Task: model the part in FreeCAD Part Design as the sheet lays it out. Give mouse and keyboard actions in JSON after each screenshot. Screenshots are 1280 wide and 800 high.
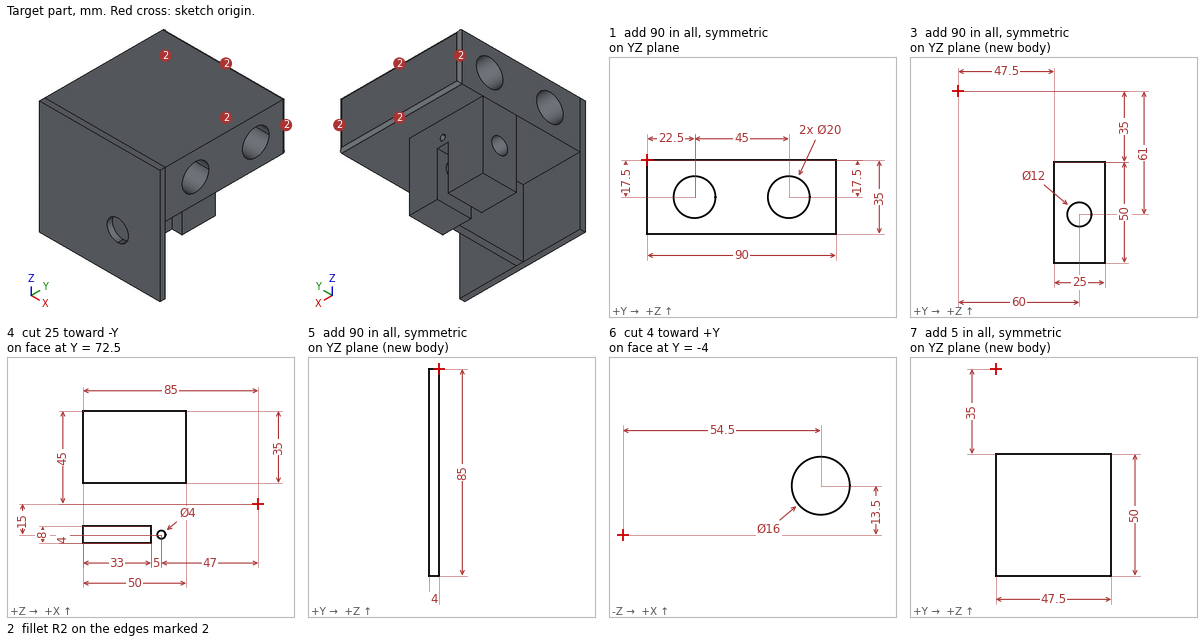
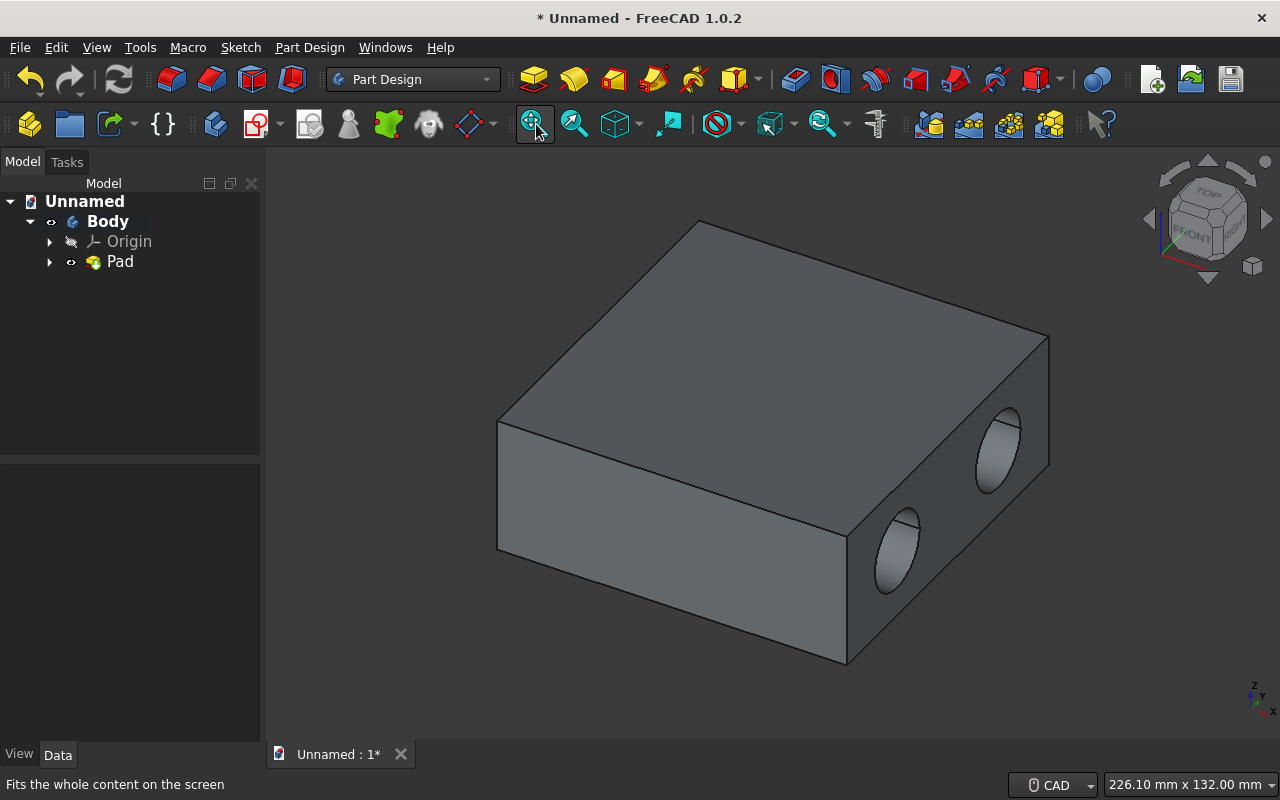
{"action": "key", "text": "0"}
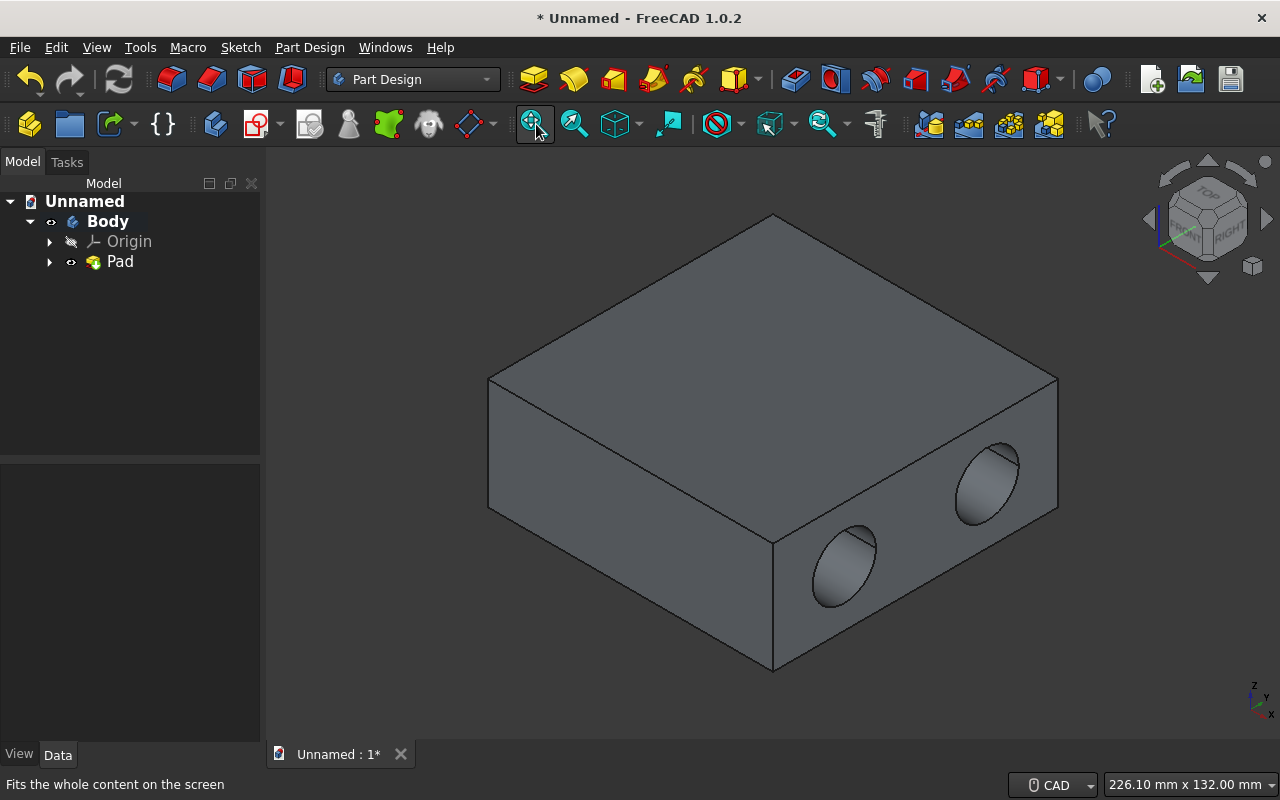
{"action": "key", "text": "2"}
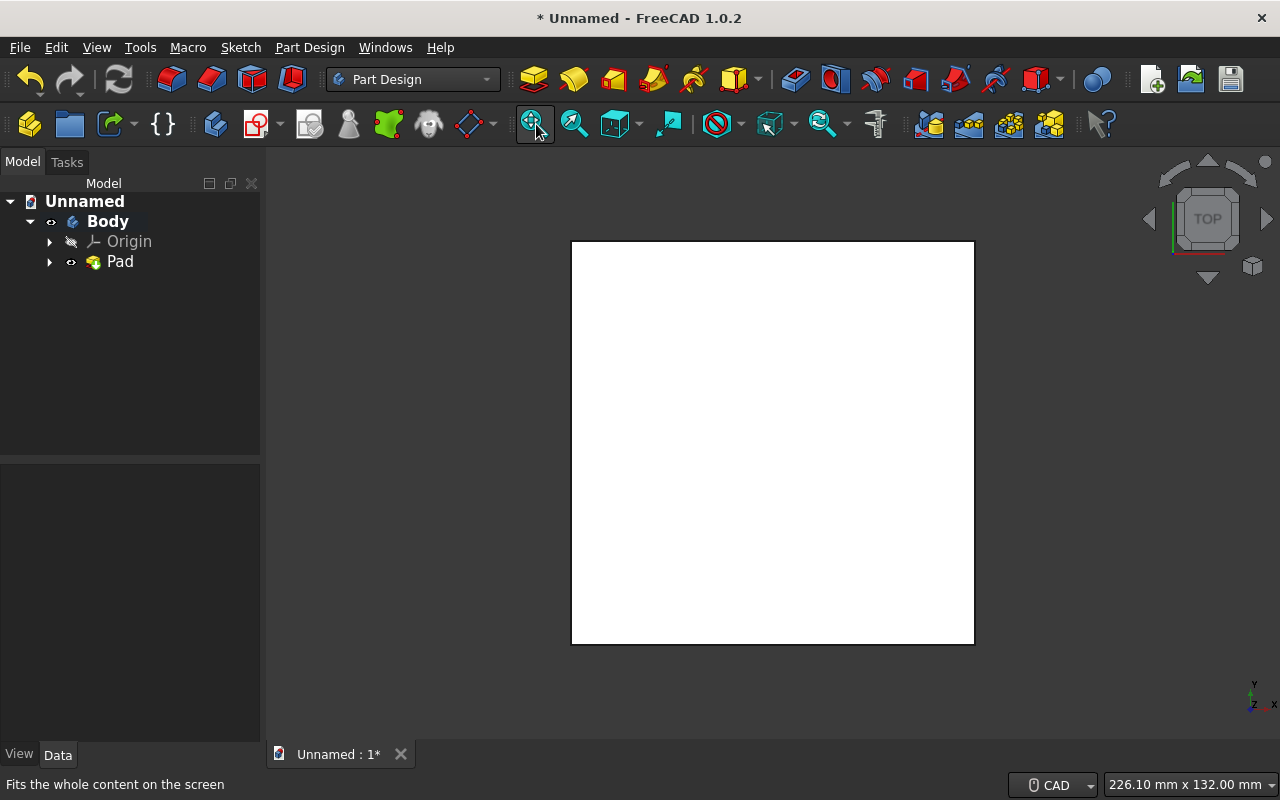
{"action": "key", "text": "1"}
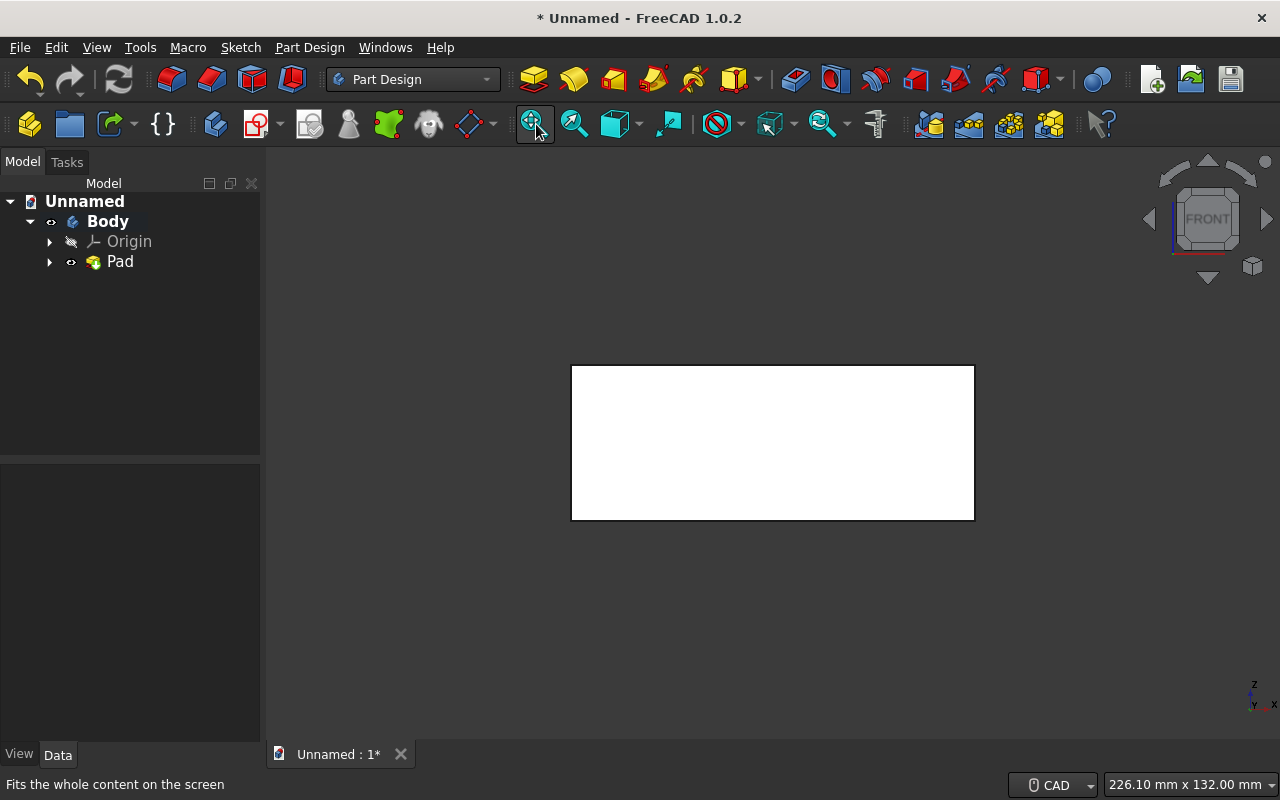
{"action": "left_click", "coordinate": [536, 124]}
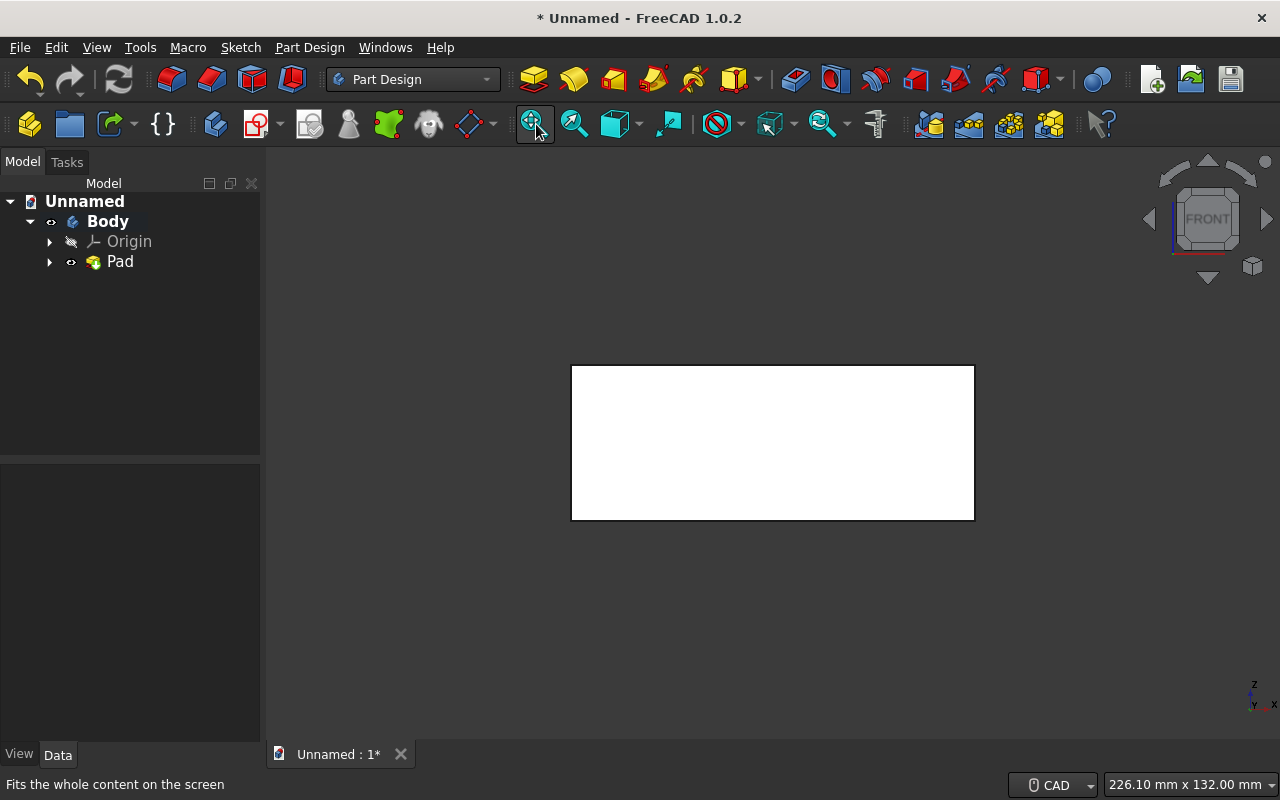
{"action": "key", "text": "3"}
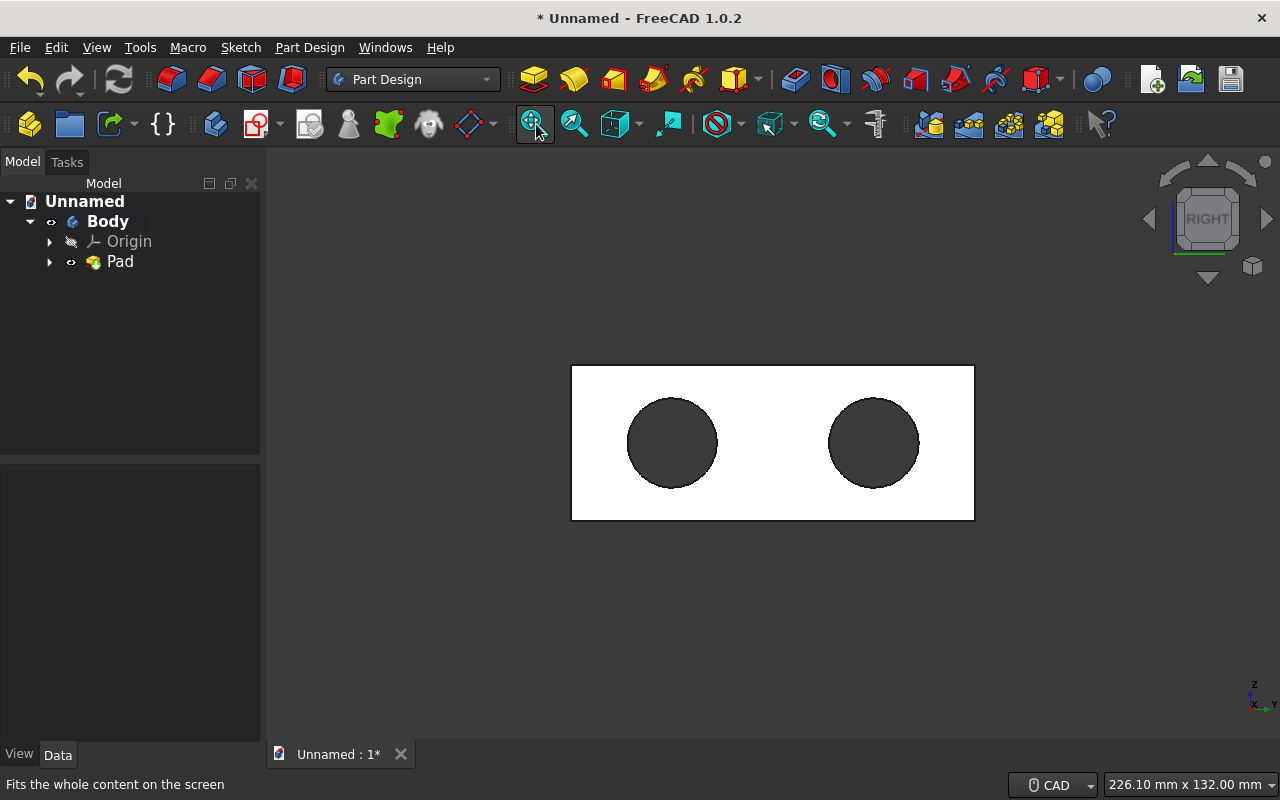
{"action": "key", "text": "v f"}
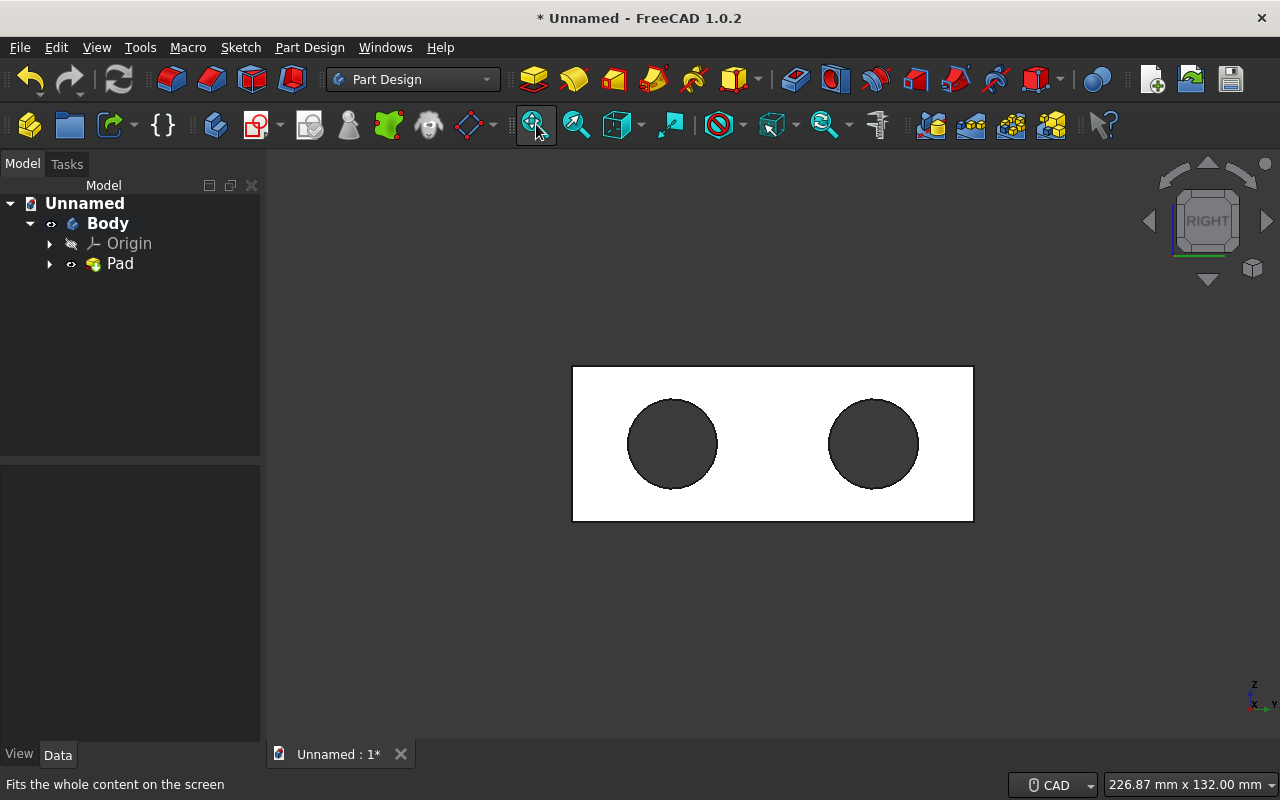
{"action": "key", "text": "5"}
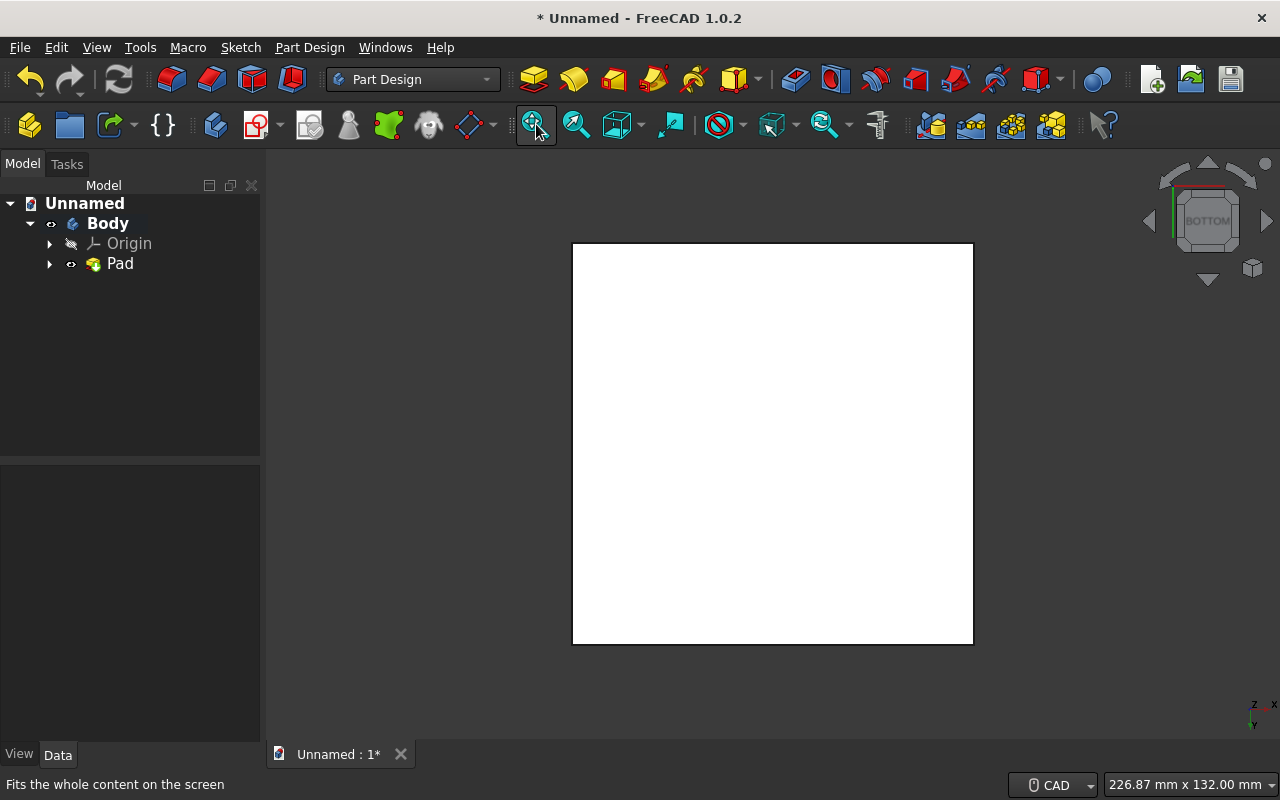
{"action": "key", "text": "4"}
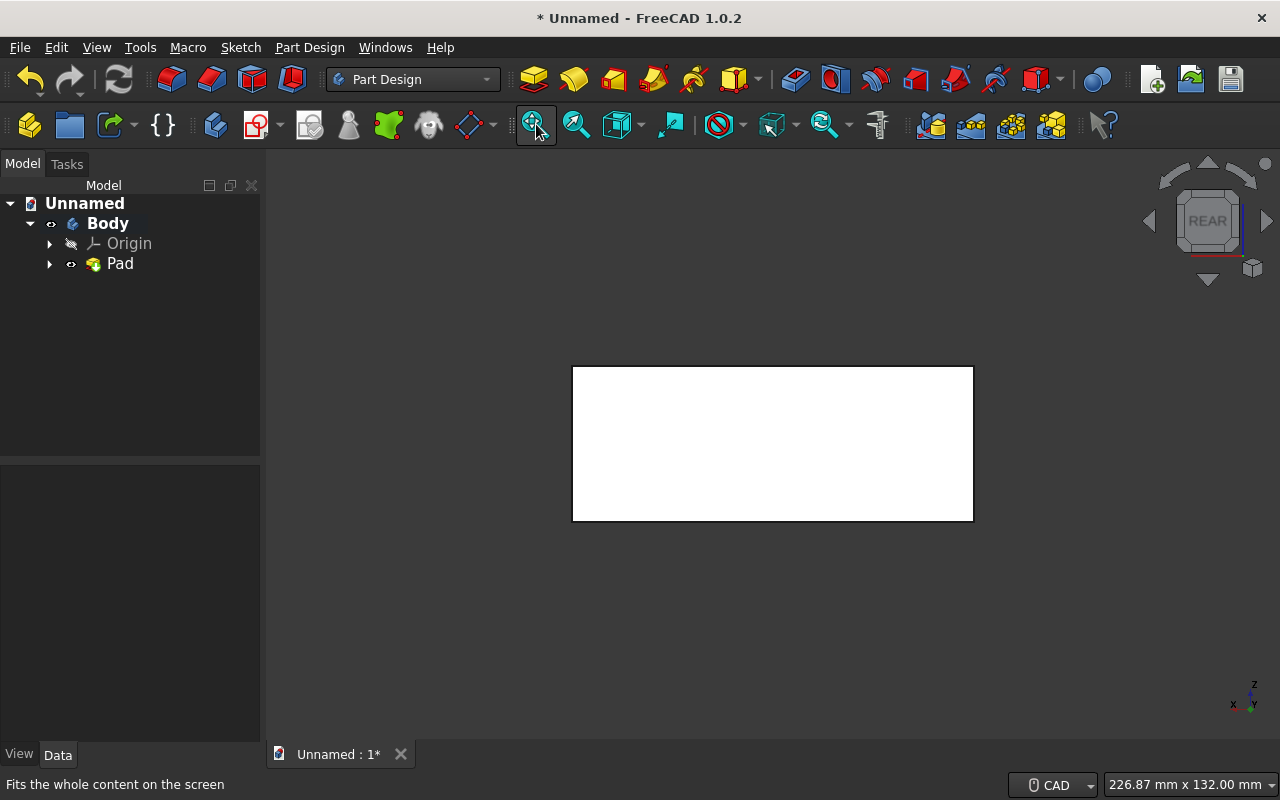
{"action": "key", "text": "v f"}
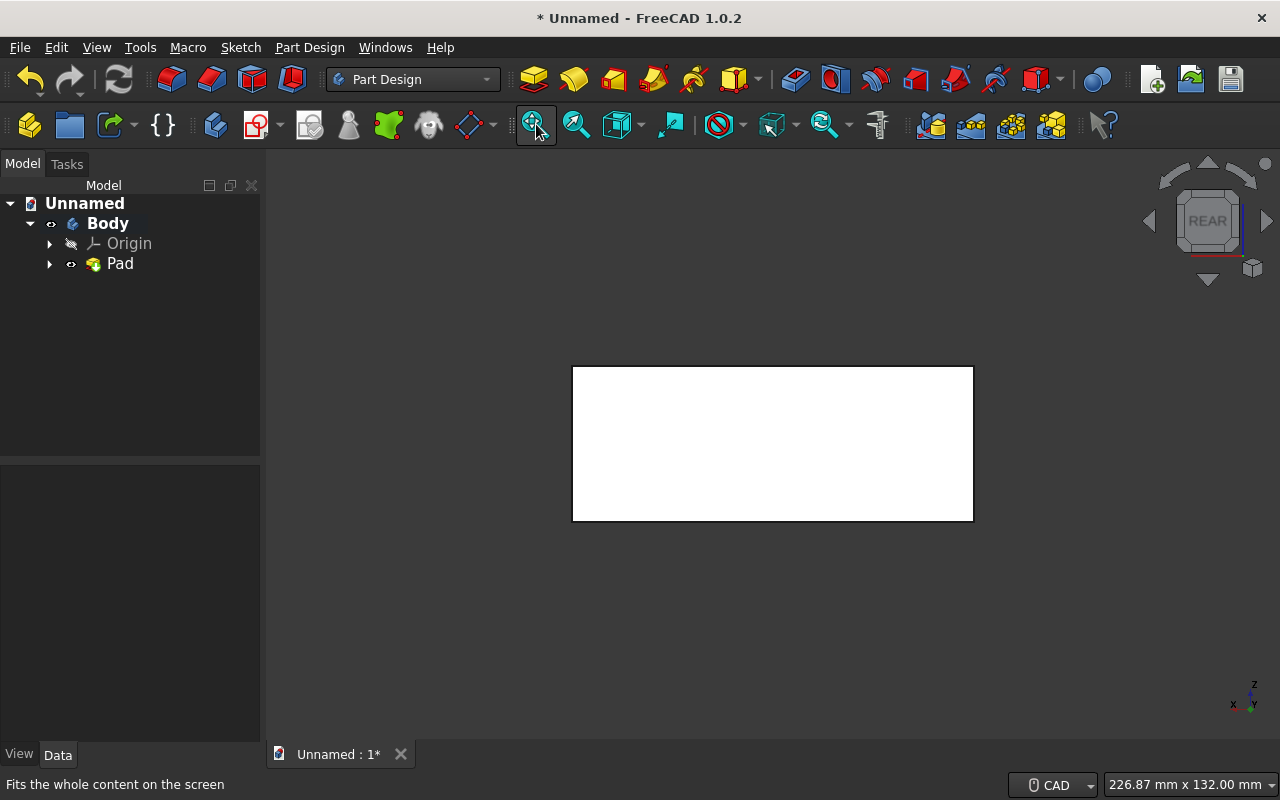
{"action": "left_click", "coordinate": [716, 443]}